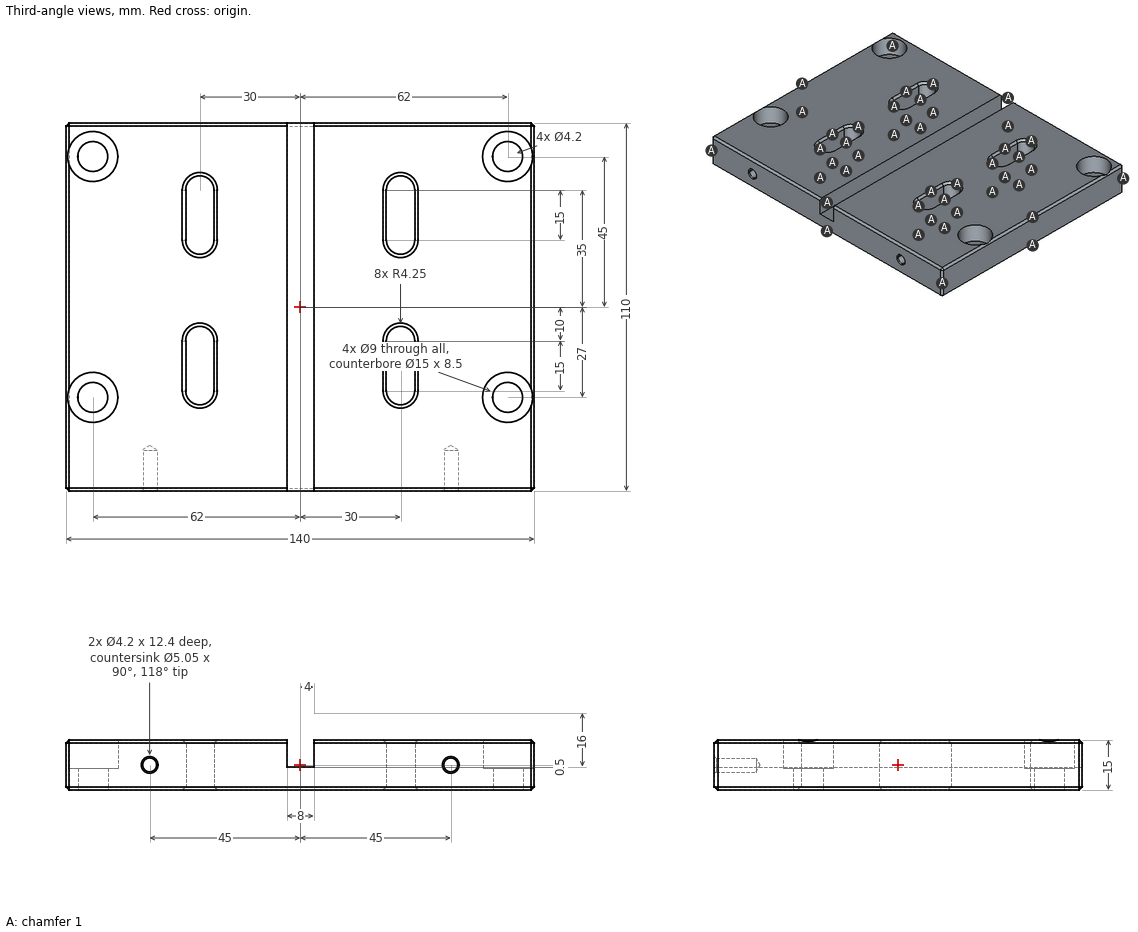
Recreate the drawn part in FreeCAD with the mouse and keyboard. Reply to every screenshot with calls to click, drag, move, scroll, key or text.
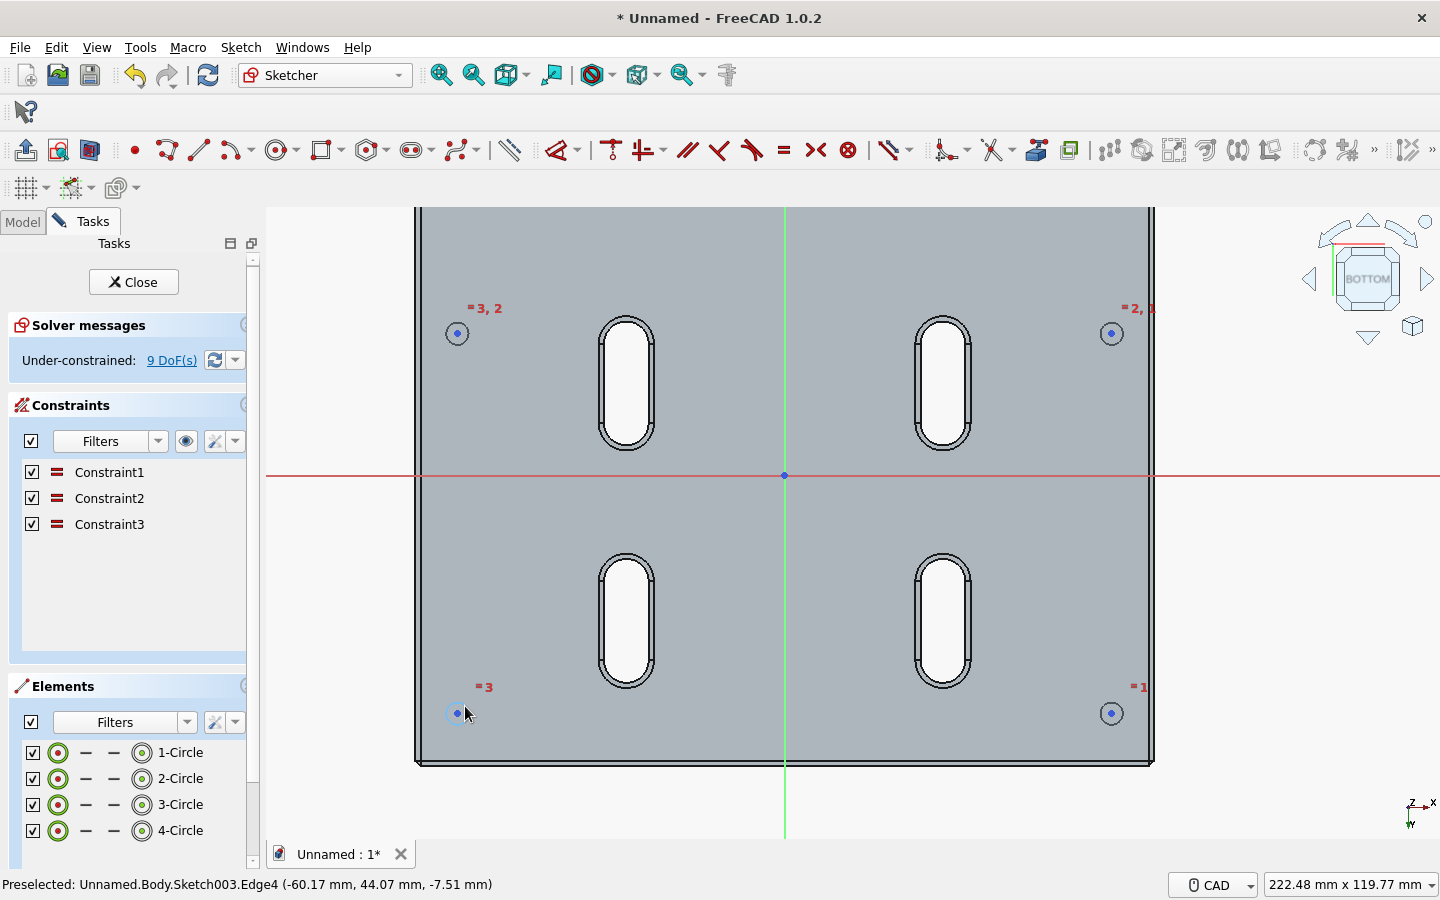
click(1112, 714)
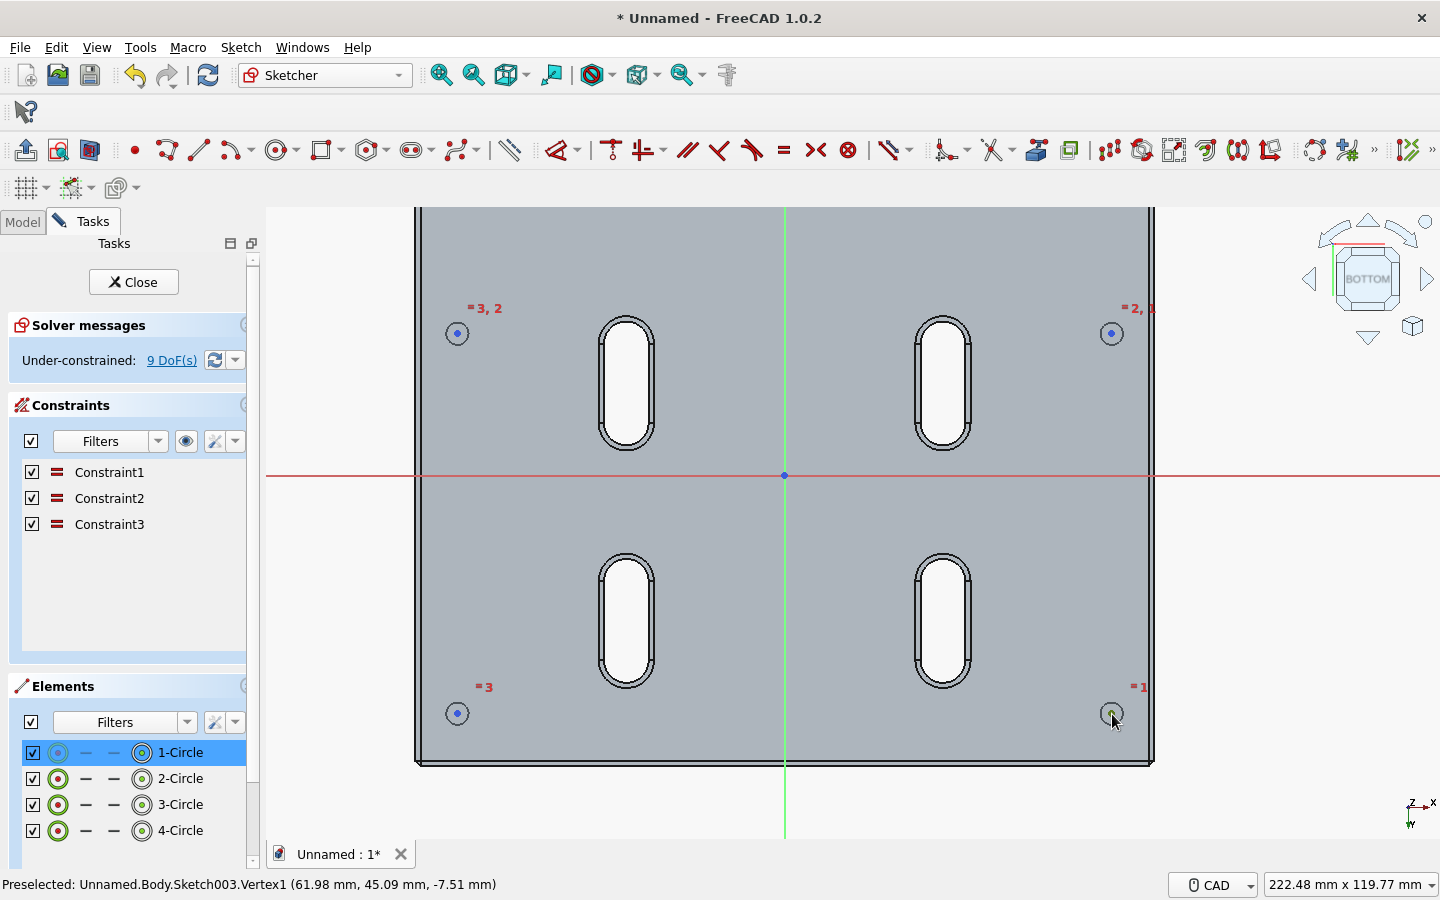
click(1112, 334)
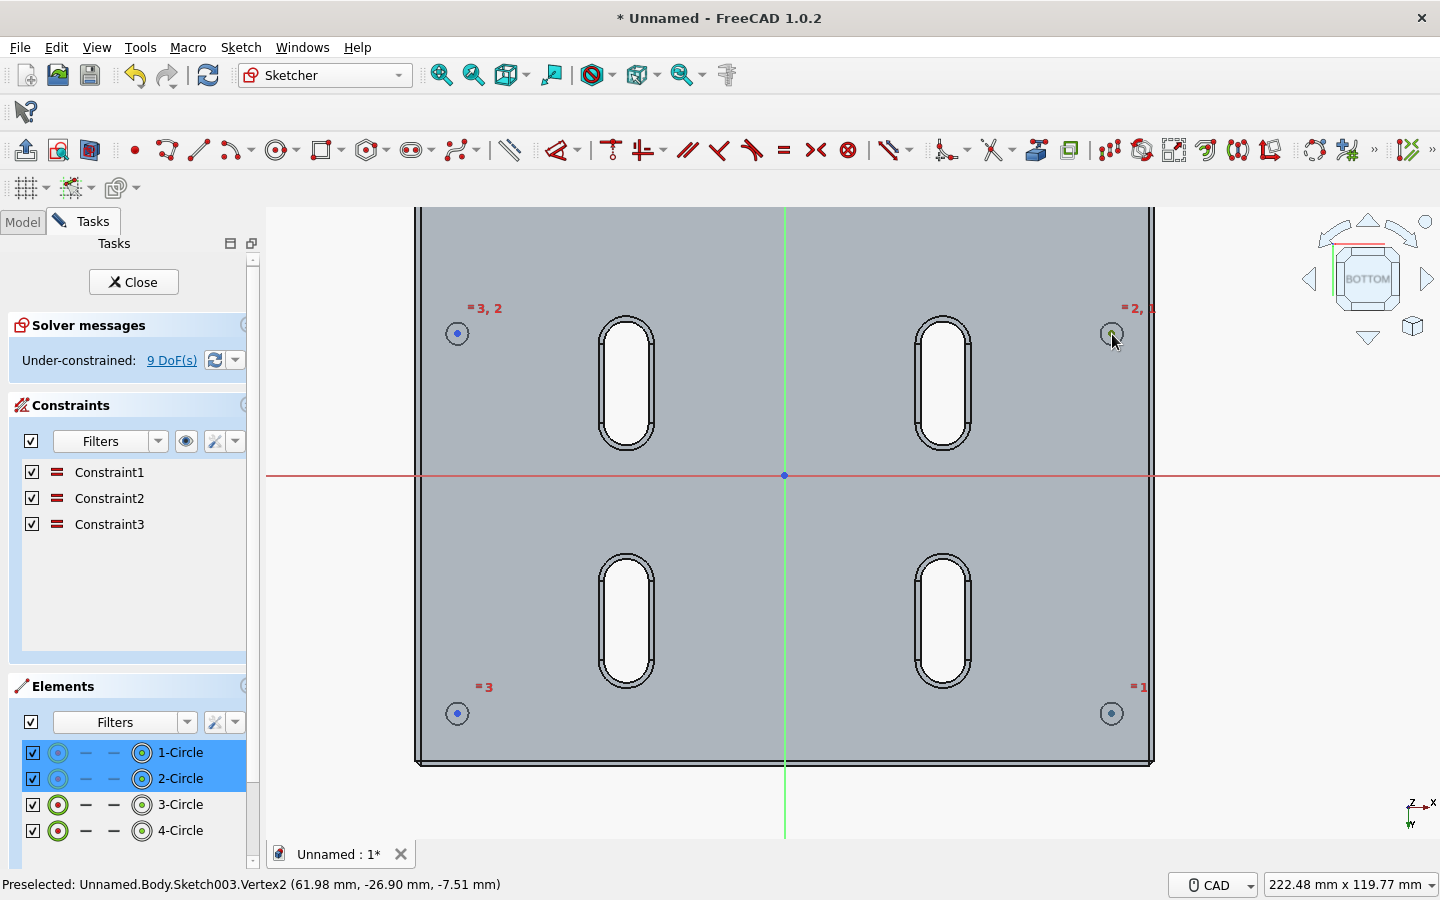
key(v)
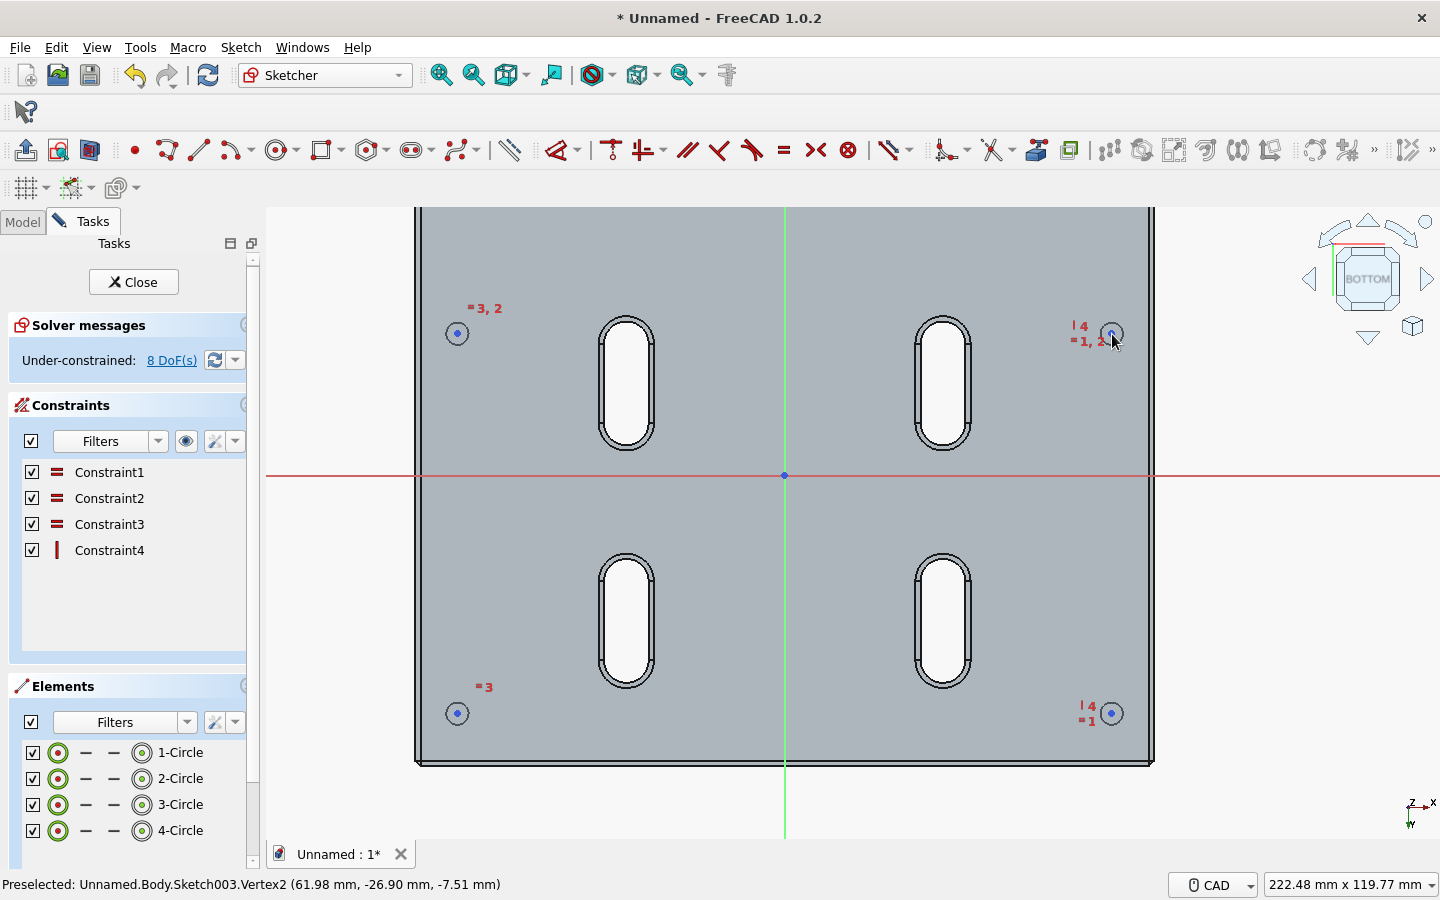
click(1112, 334)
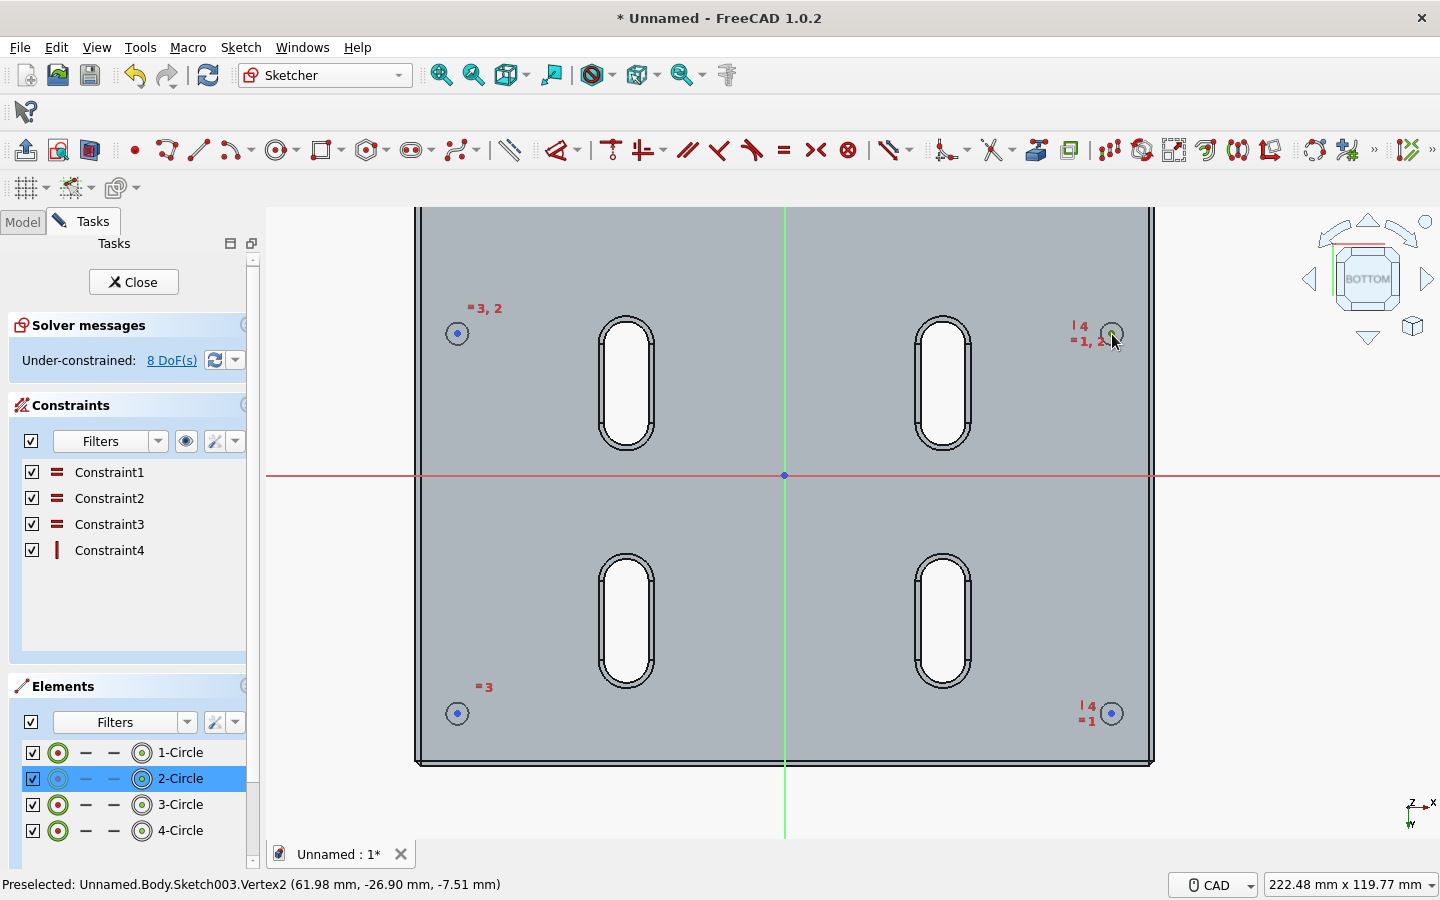
click(457, 334)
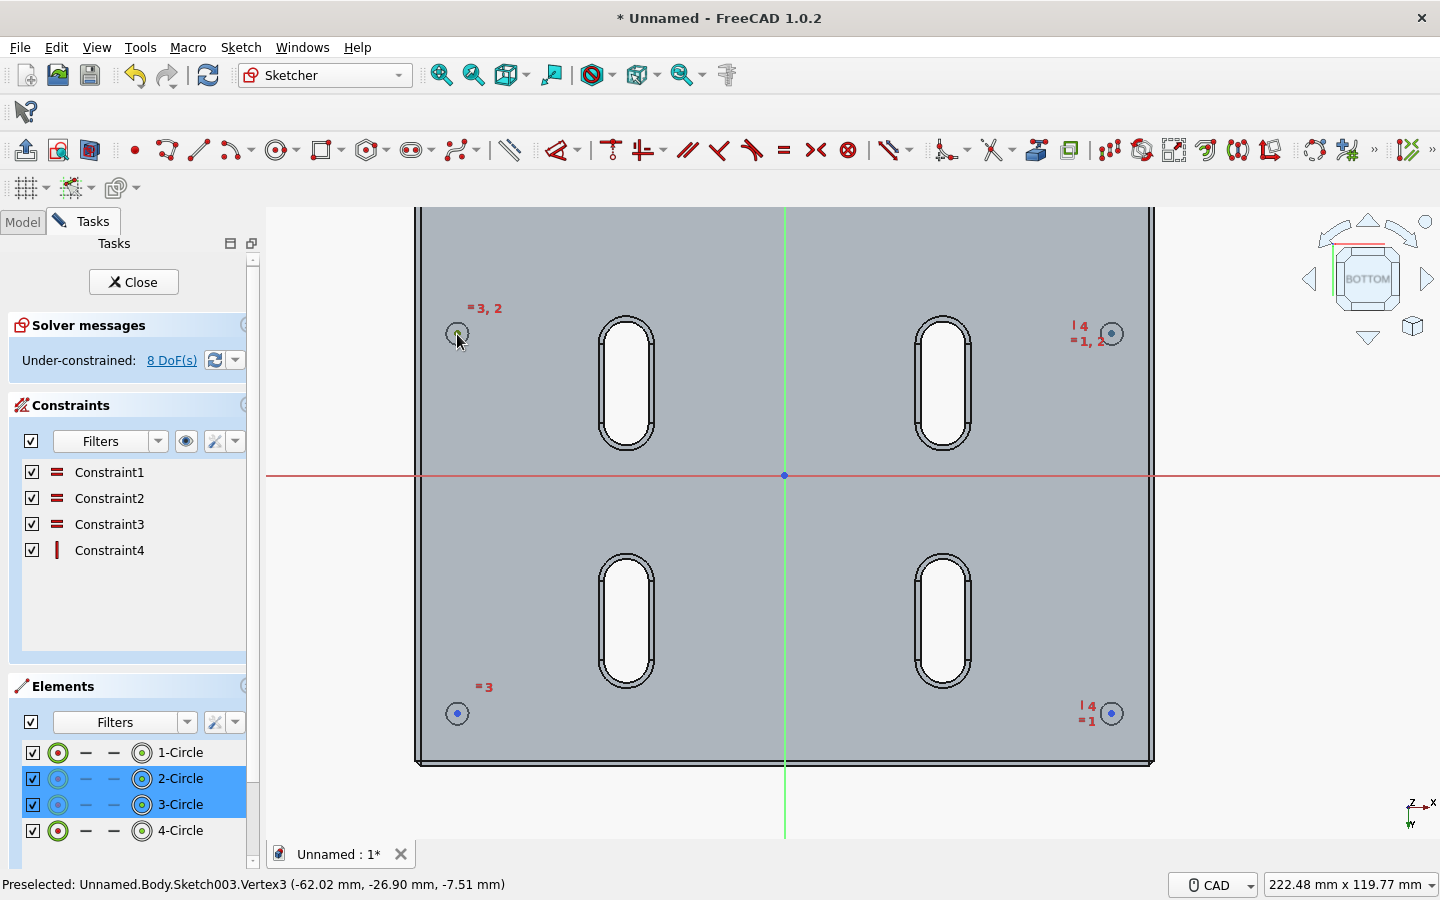
key(h)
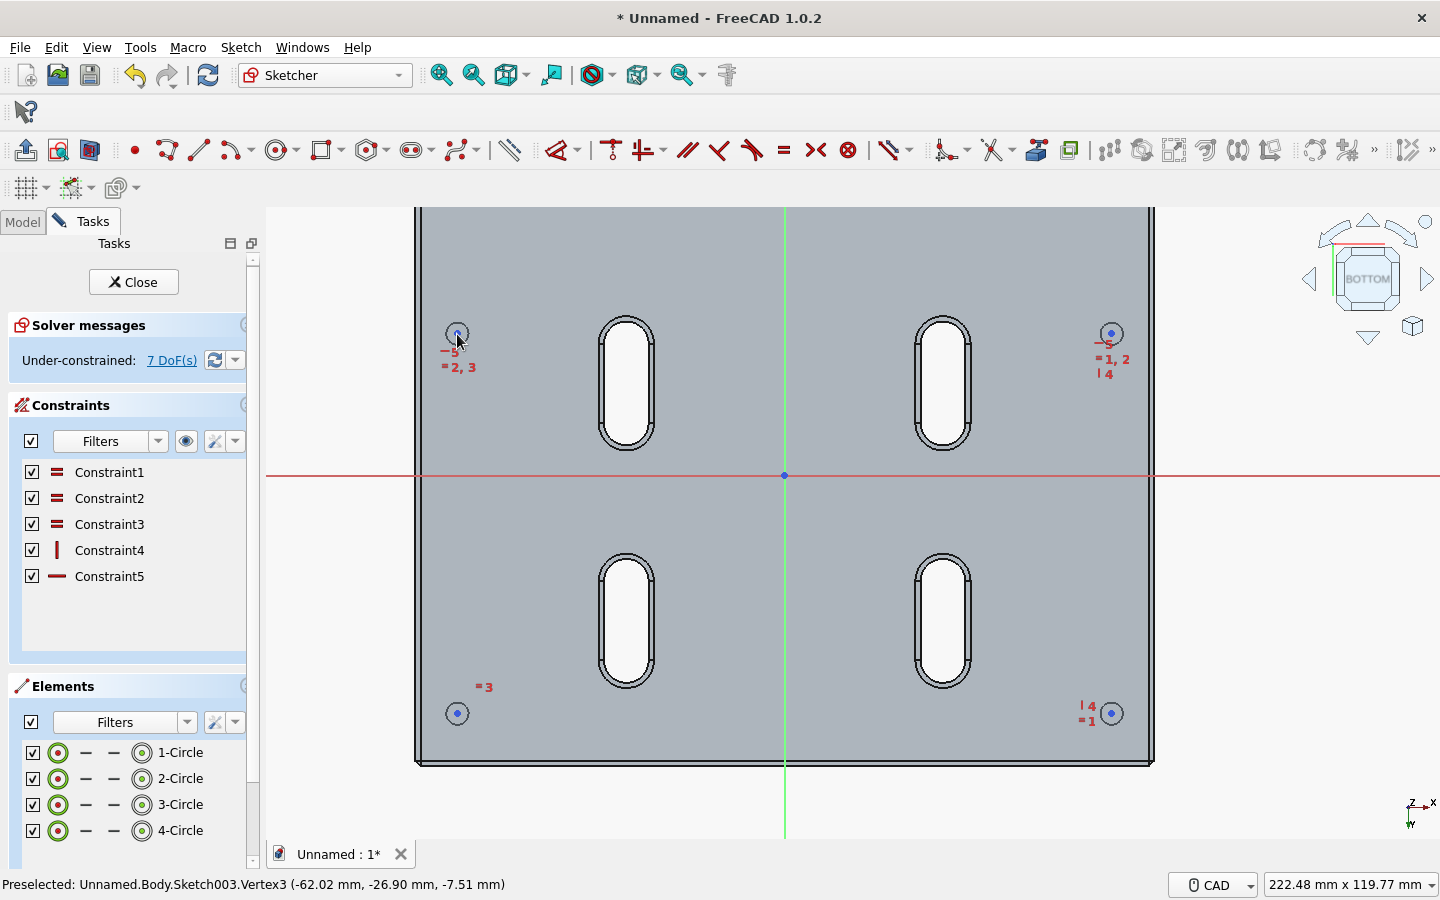
click(457, 334)